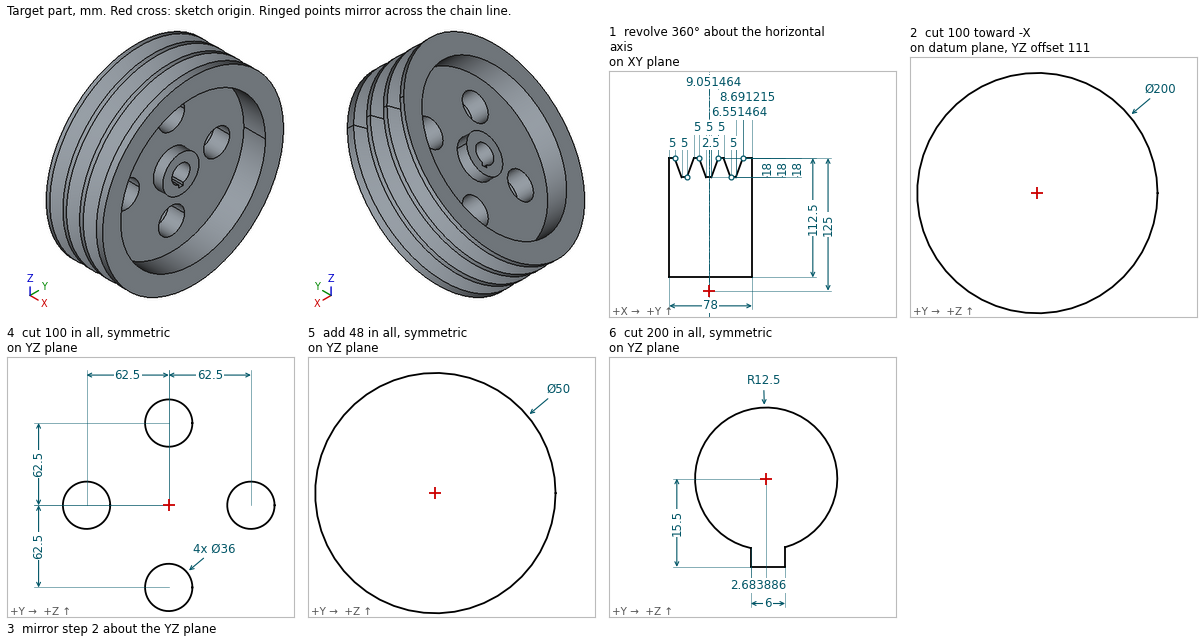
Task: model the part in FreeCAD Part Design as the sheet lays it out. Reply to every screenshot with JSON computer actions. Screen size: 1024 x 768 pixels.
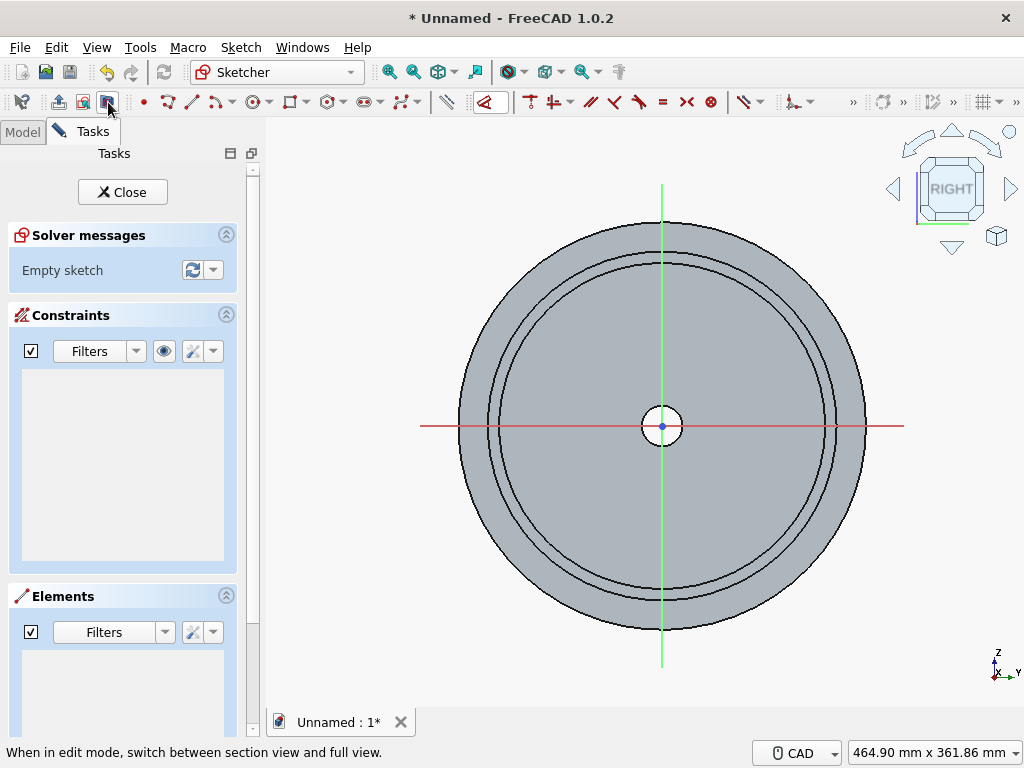
{"action": "scroll", "coordinate": [836, 455], "scroll_direction": "up", "scroll_amount": 2}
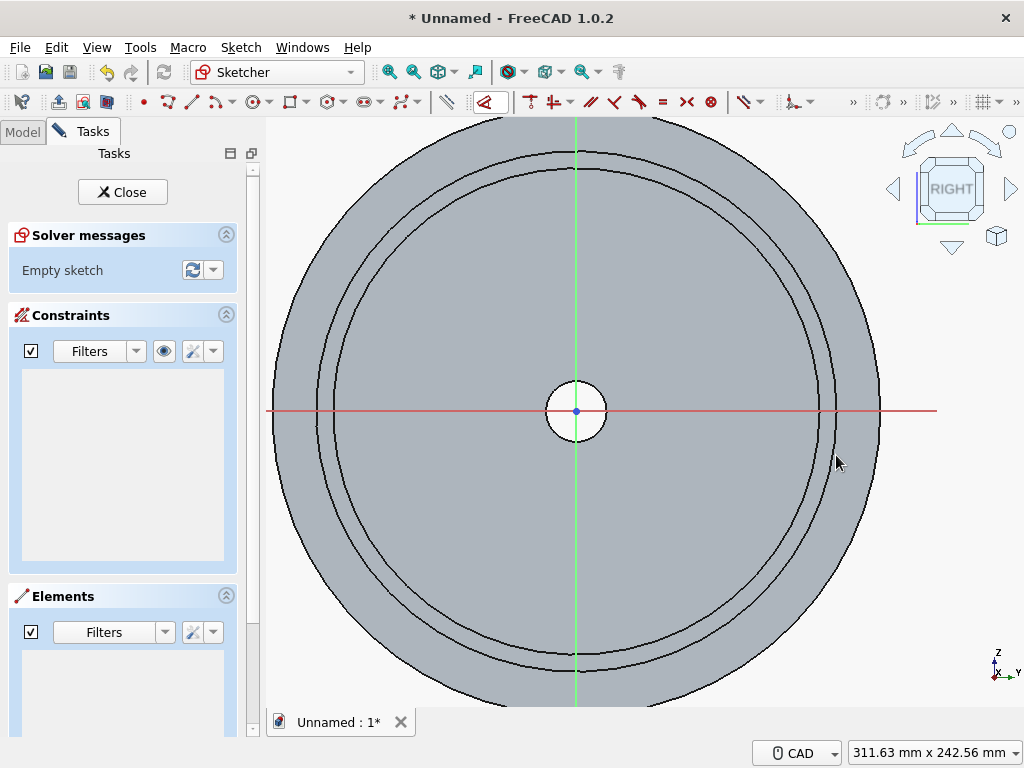
{"action": "left_click", "coordinate": [254, 102]}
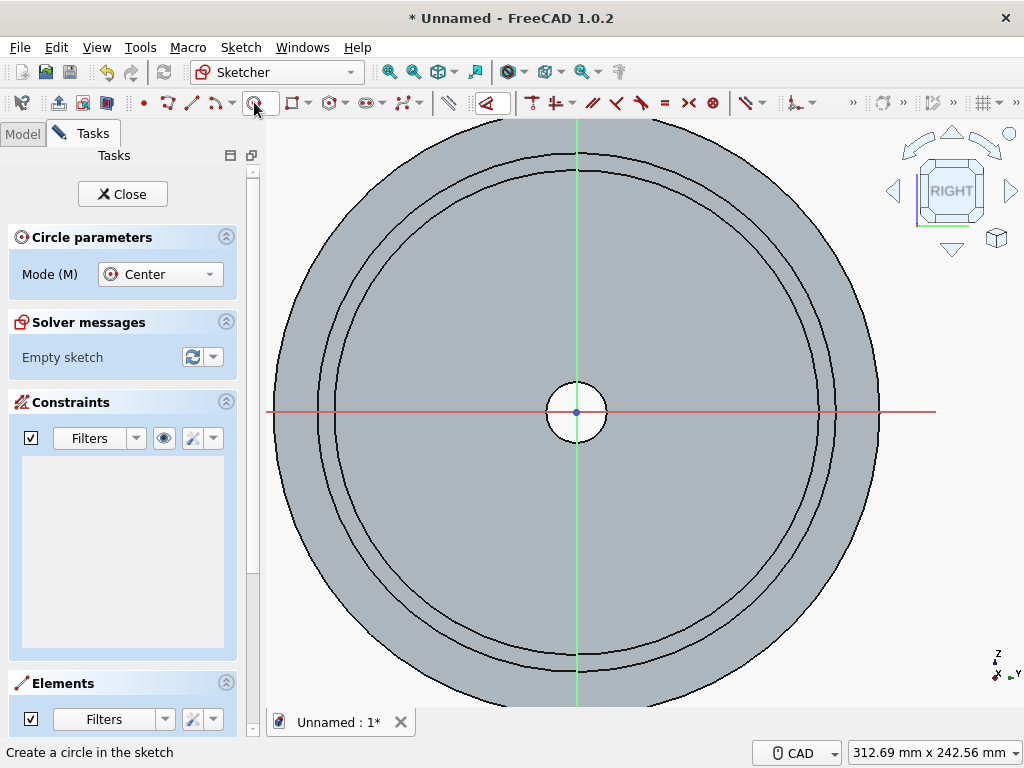
{"action": "left_click", "coordinate": [577, 564]}
{"action": "left_click", "coordinate": [607, 533]}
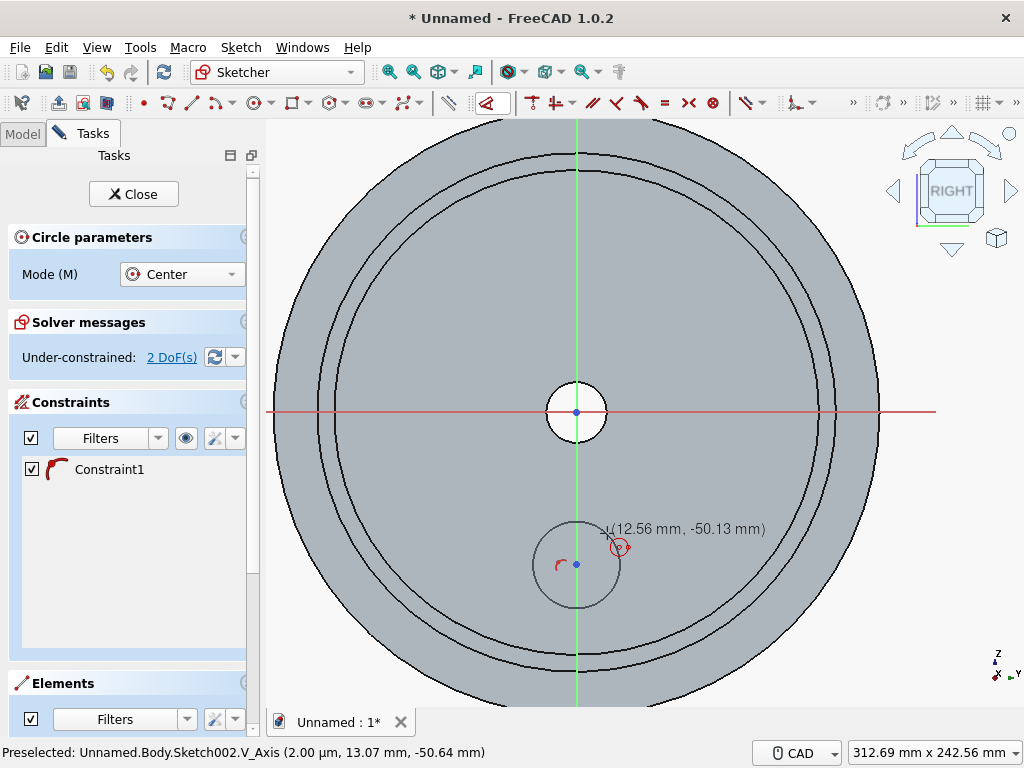
{"action": "left_click", "coordinate": [425, 412]}
{"action": "left_click", "coordinate": [456, 382]}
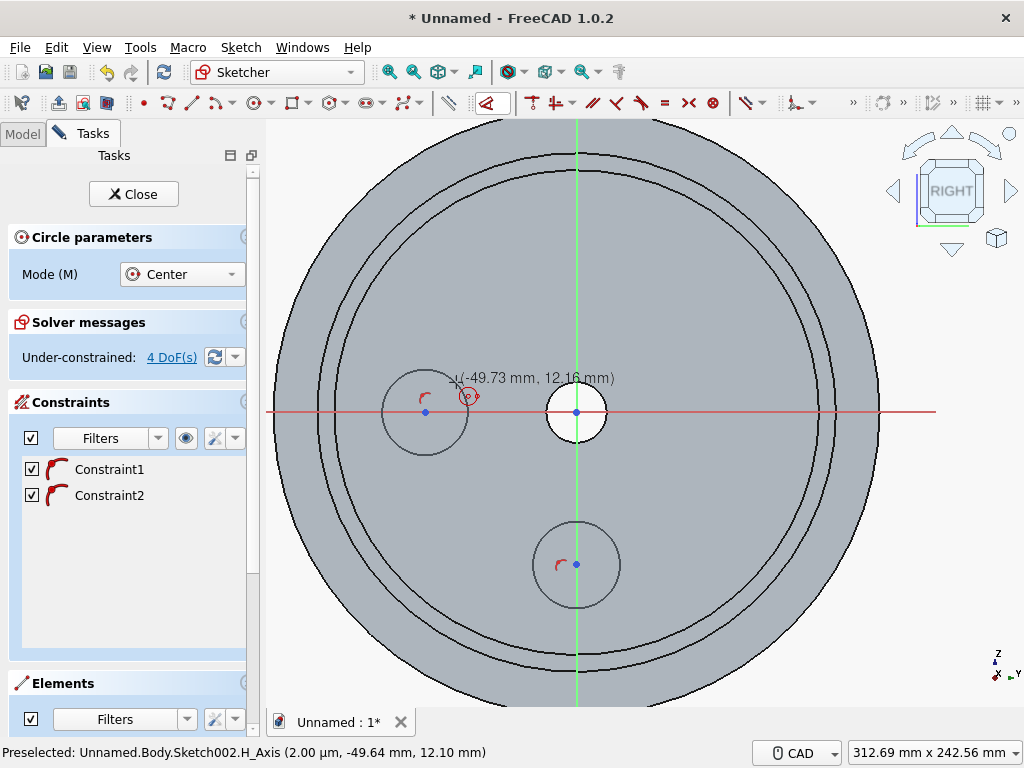
{"action": "left_click", "coordinate": [577, 261]}
{"action": "left_click", "coordinate": [607, 230]}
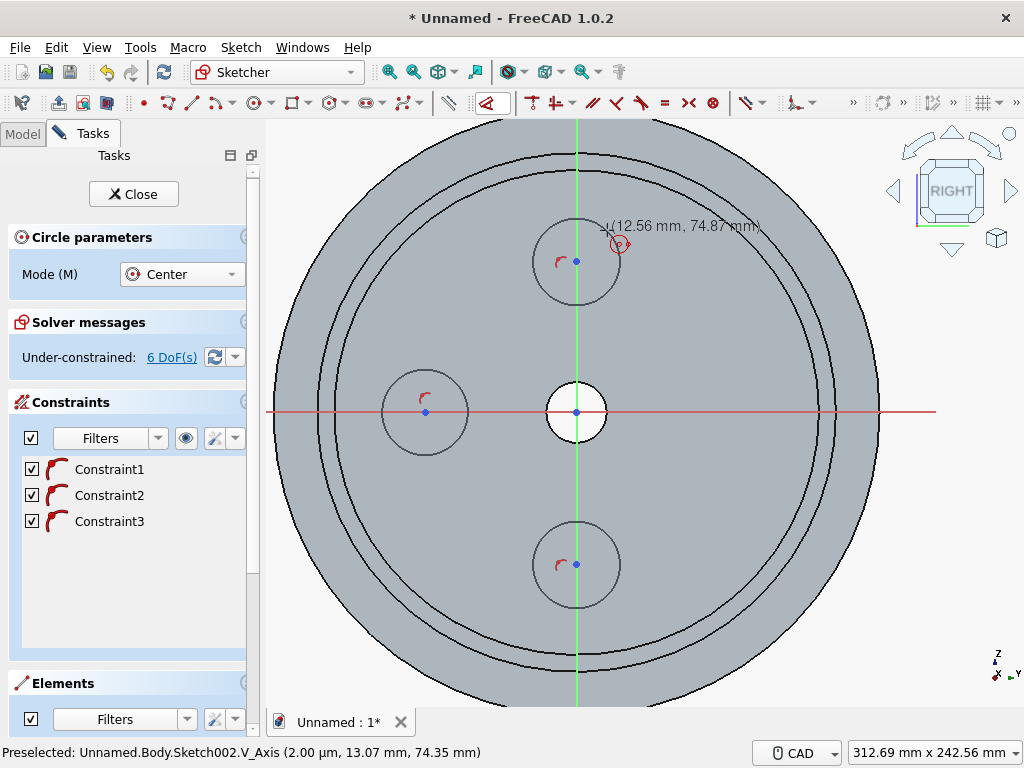
{"action": "left_click", "coordinate": [728, 412]}
{"action": "left_click", "coordinate": [759, 382]}
{"action": "key", "text": "Escape"}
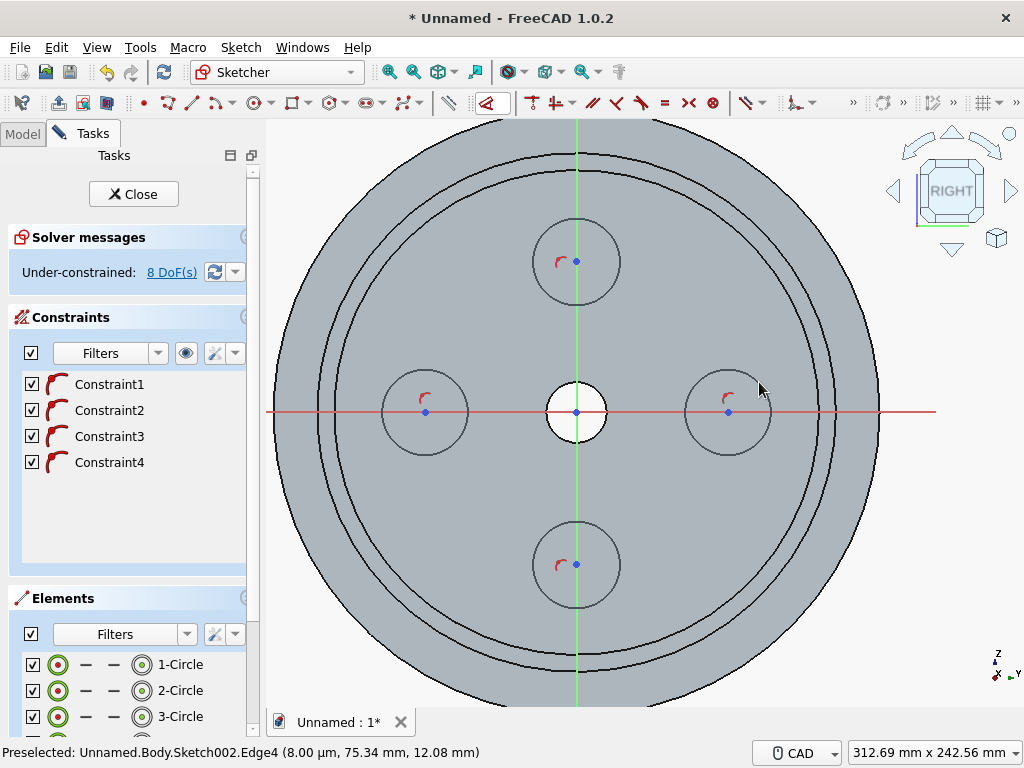
{"action": "left_click", "coordinate": [607, 534]}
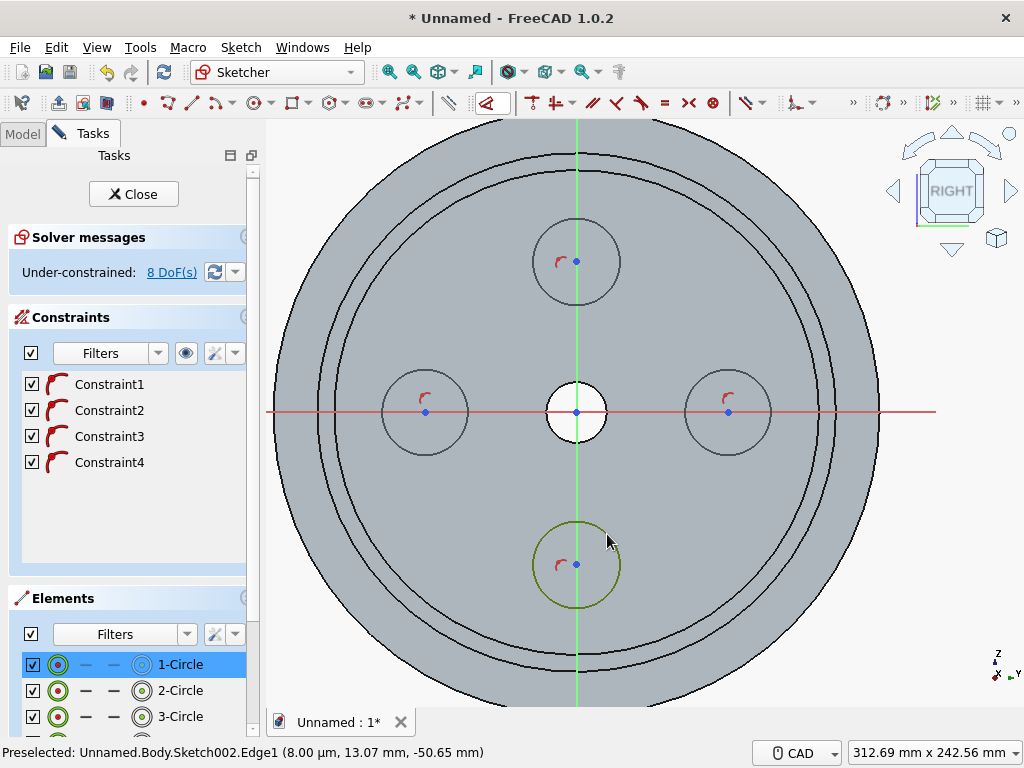
{"action": "left_click", "coordinate": [455, 382]}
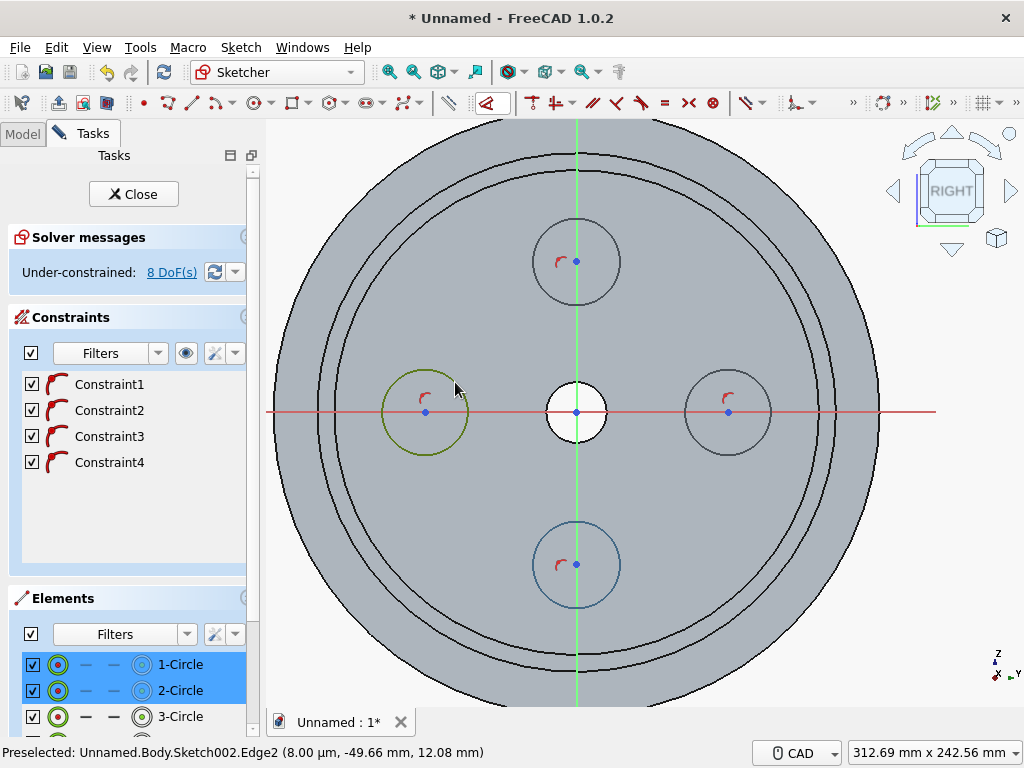
{"action": "left_click", "coordinate": [607, 231]}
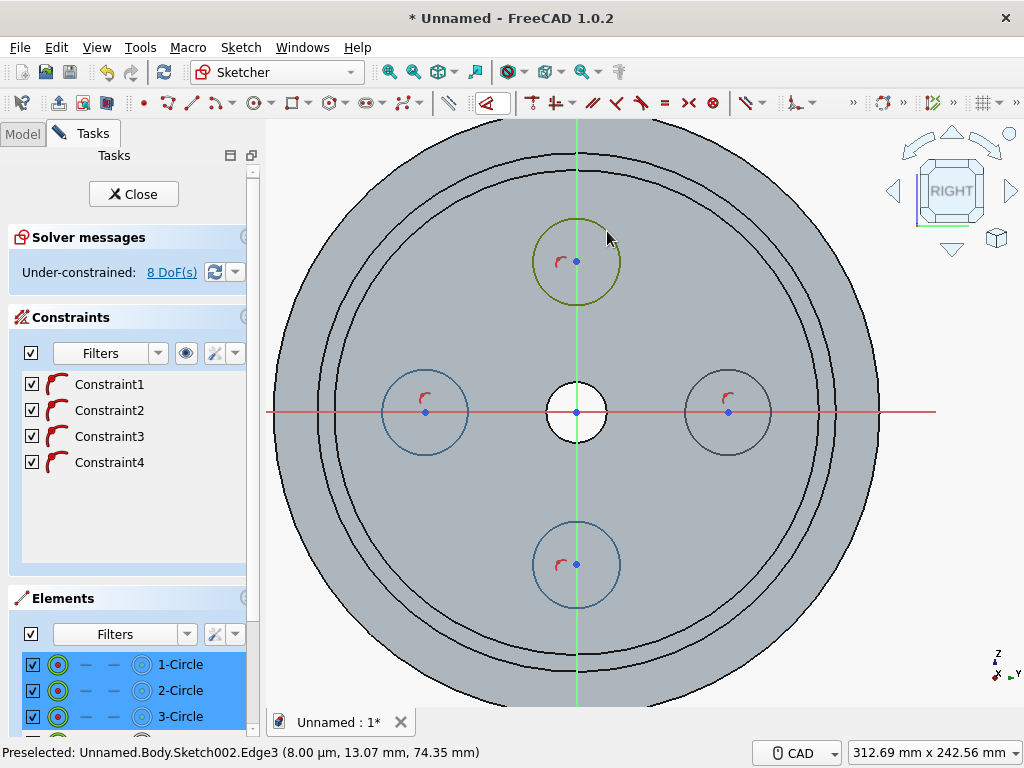
{"action": "left_click", "coordinate": [758, 382]}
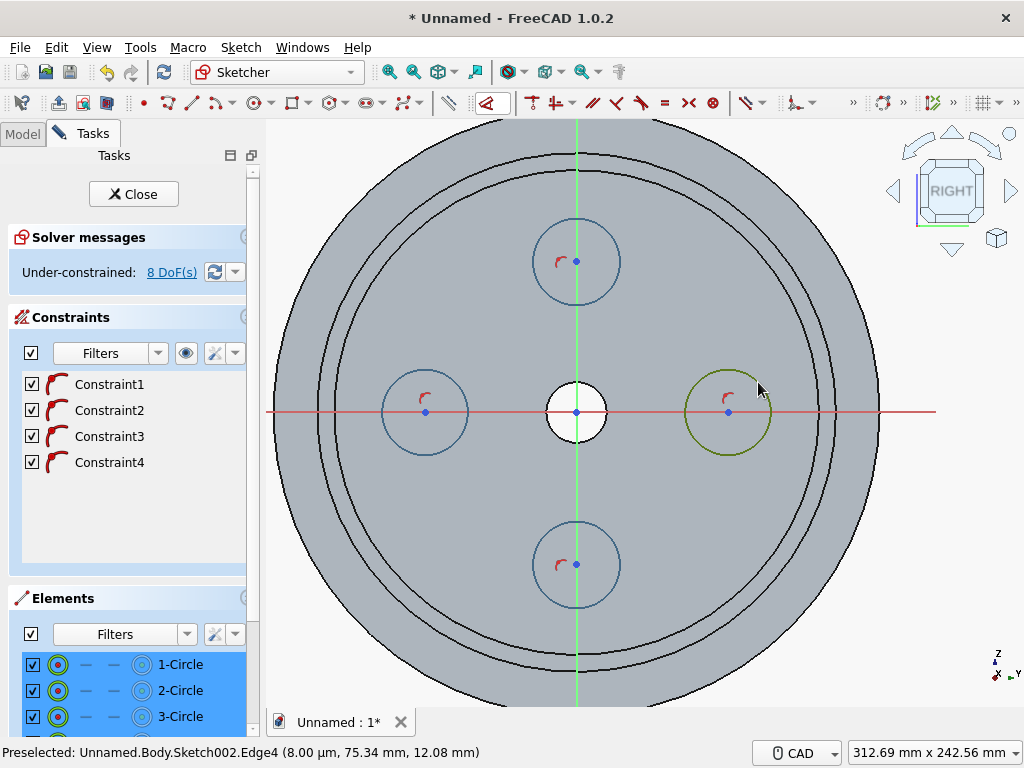
{"action": "left_click", "coordinate": [666, 104]}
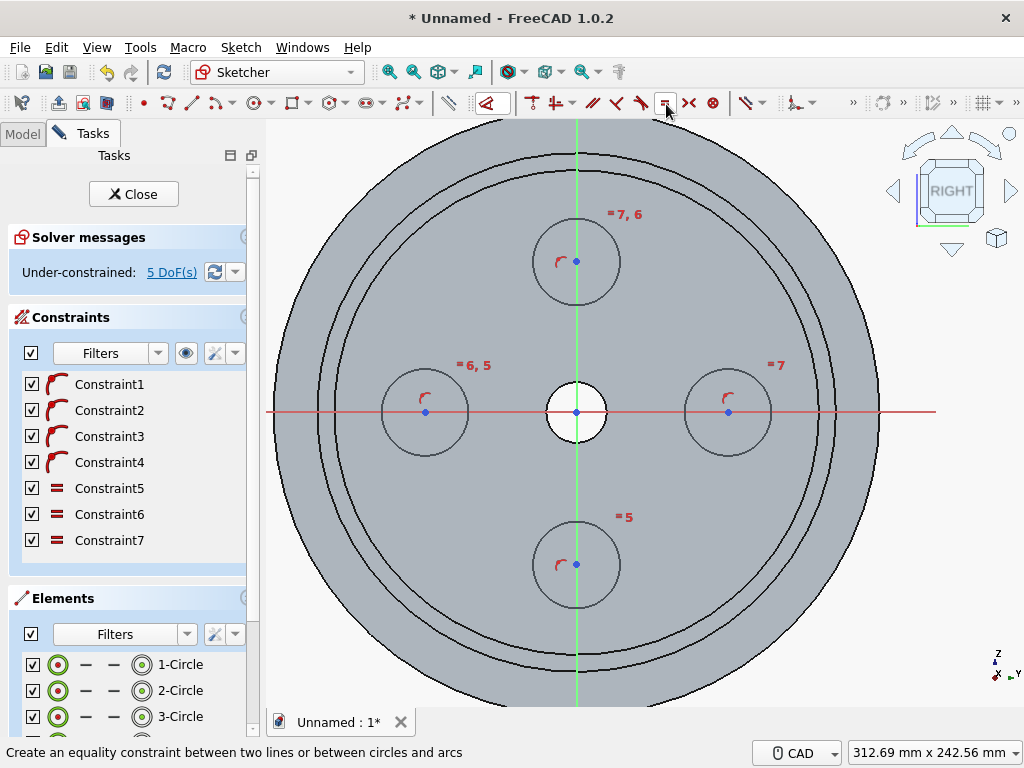
{"action": "left_click", "coordinate": [607, 534]}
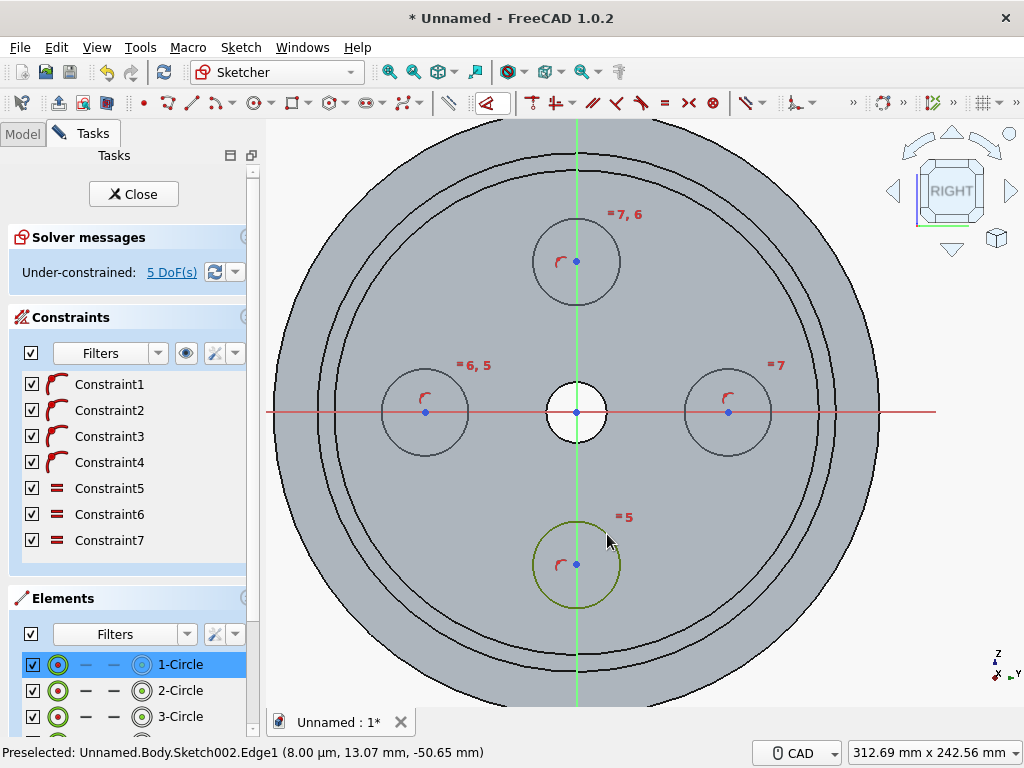
{"action": "left_click", "coordinate": [504, 104]}